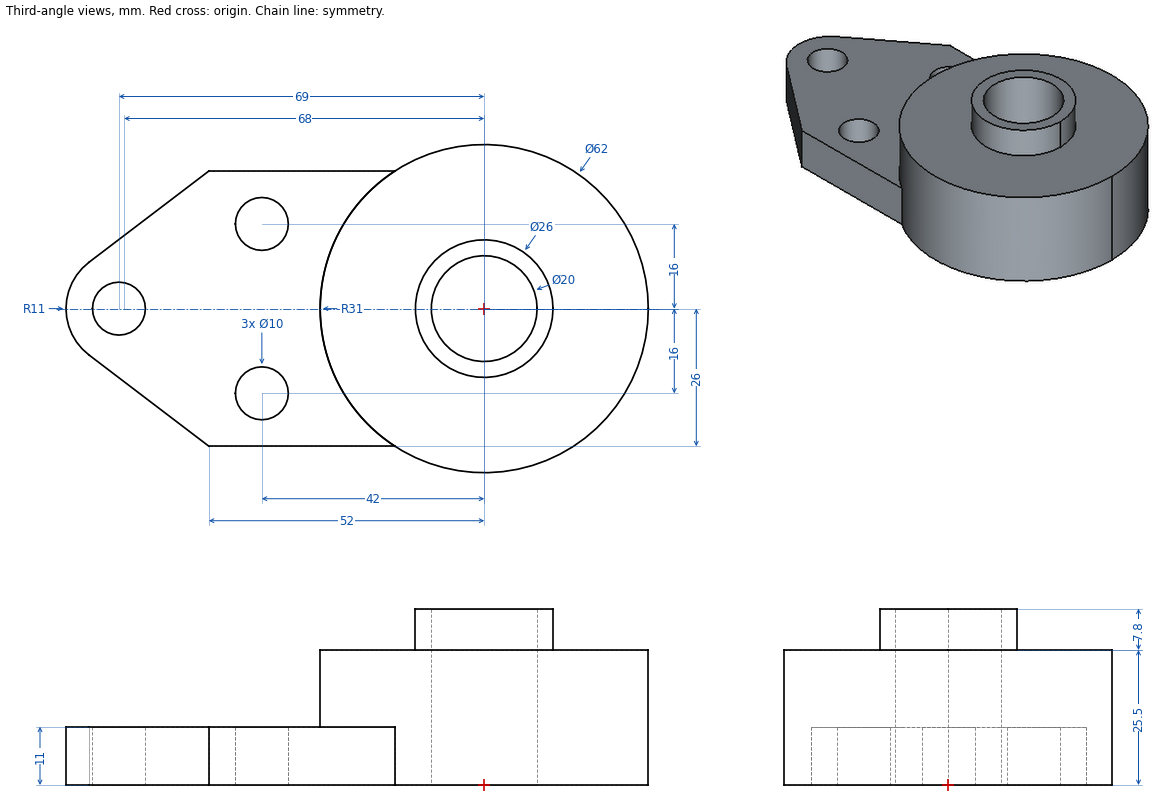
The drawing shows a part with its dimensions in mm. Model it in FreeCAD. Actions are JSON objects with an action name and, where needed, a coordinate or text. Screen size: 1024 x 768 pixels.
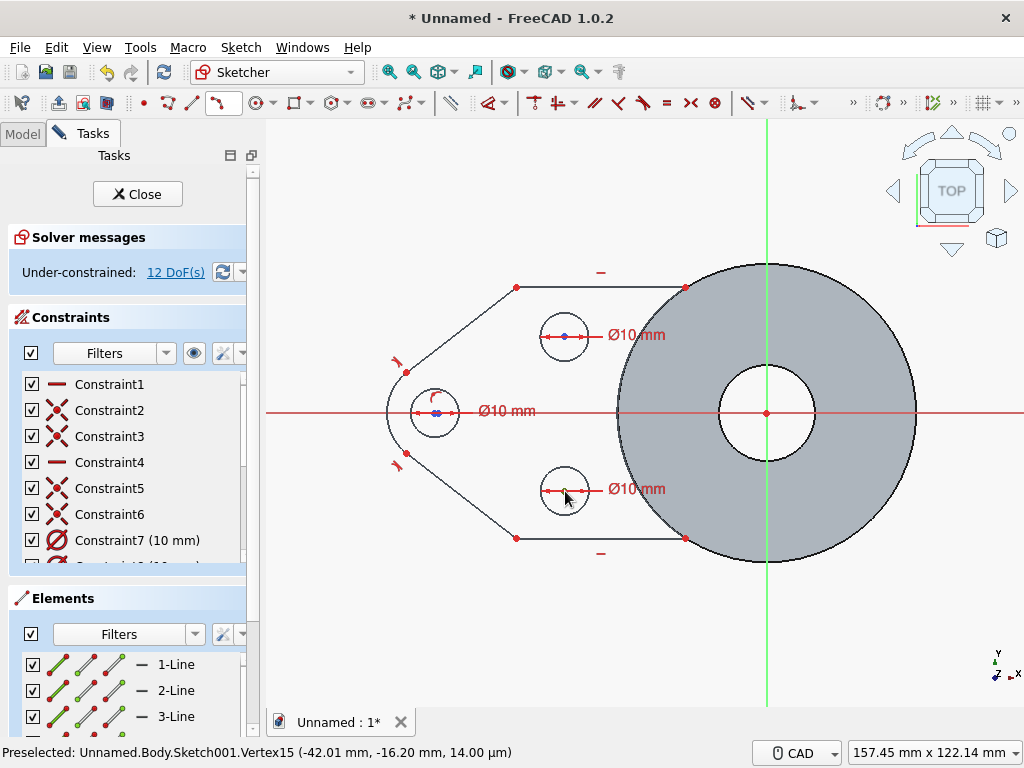
{"action": "left_click", "coordinate": [564, 337]}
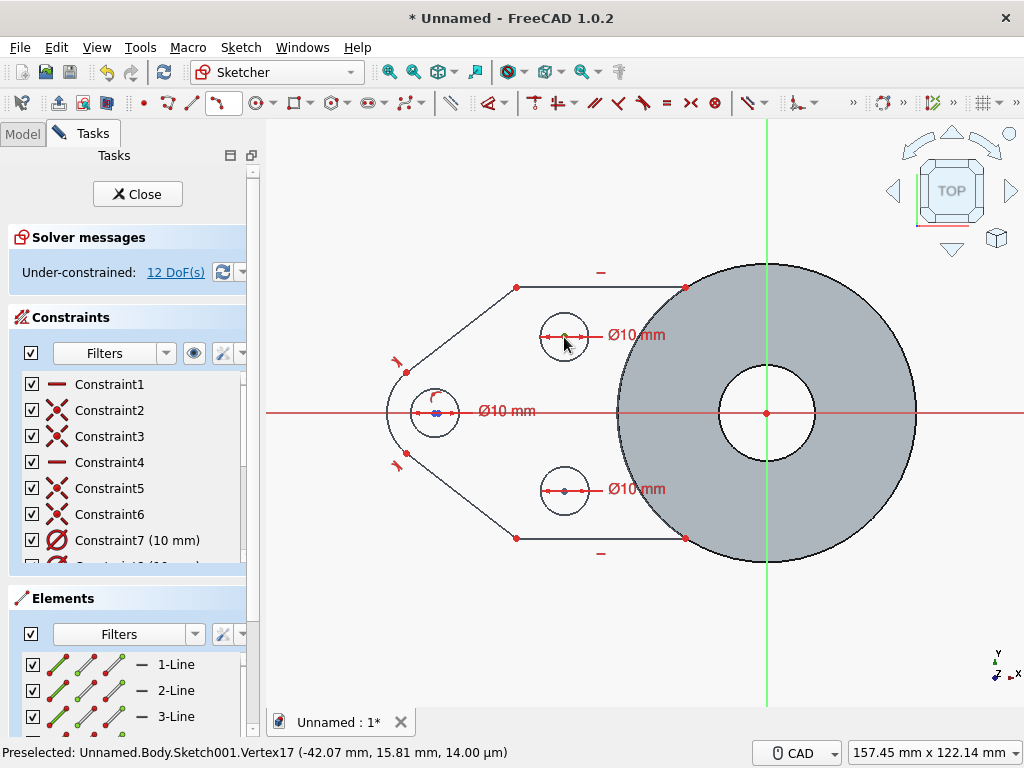
{"action": "key", "text": "v"}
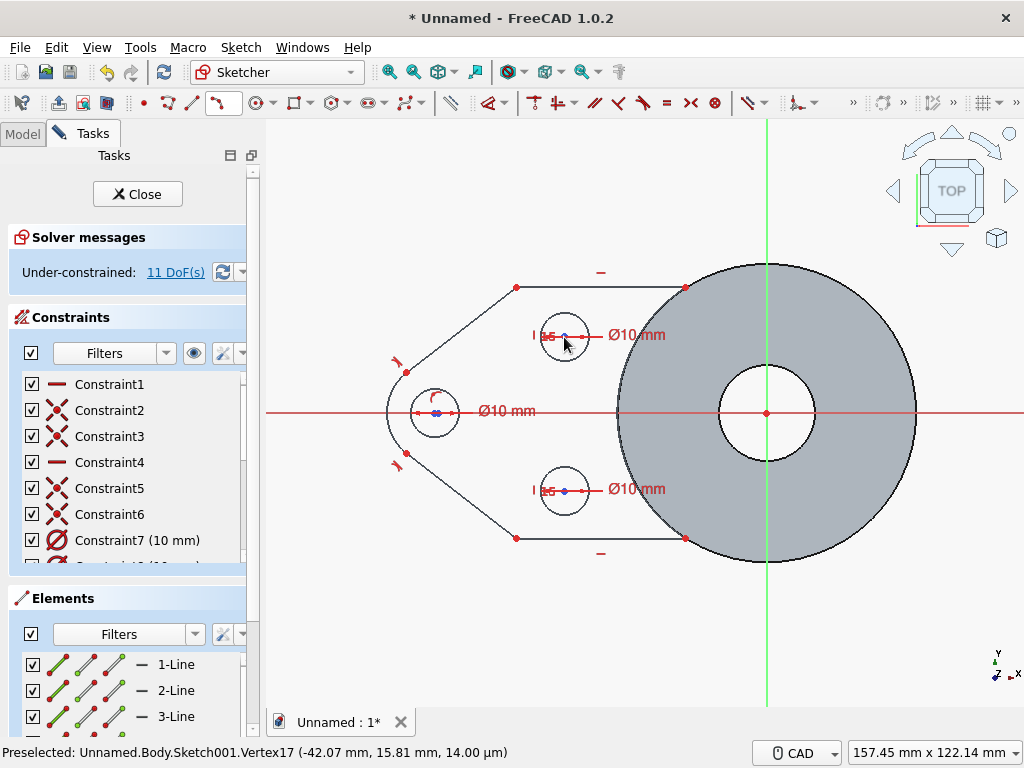
{"action": "left_click", "coordinate": [516, 539]}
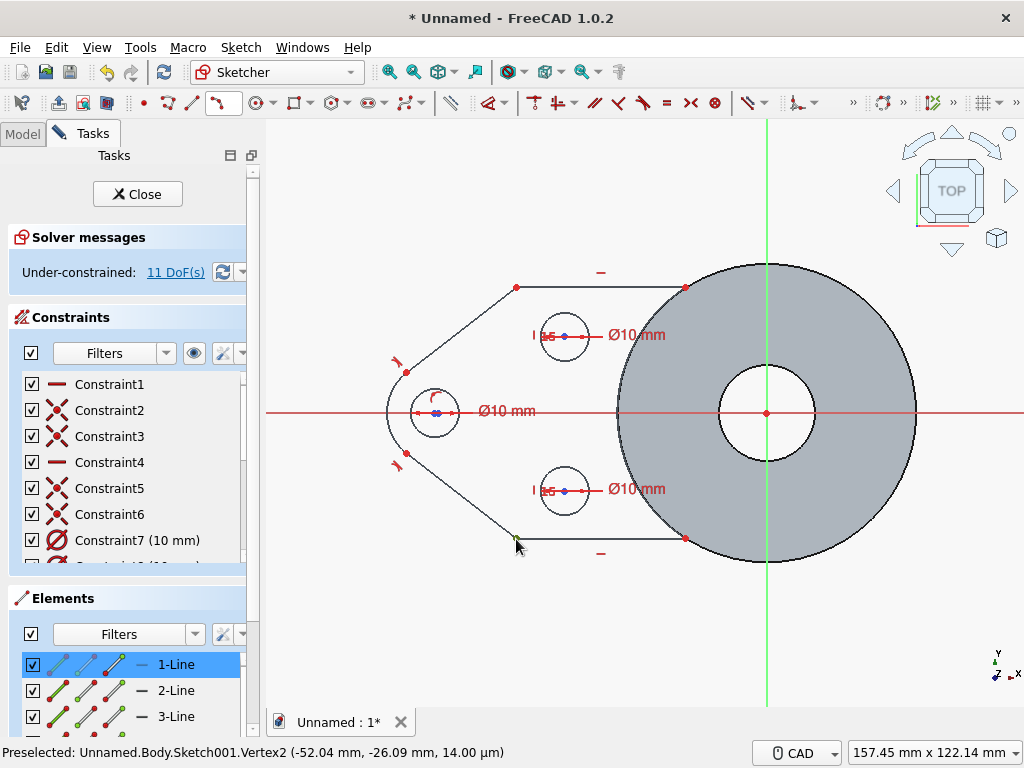
{"action": "left_click", "coordinate": [516, 287]}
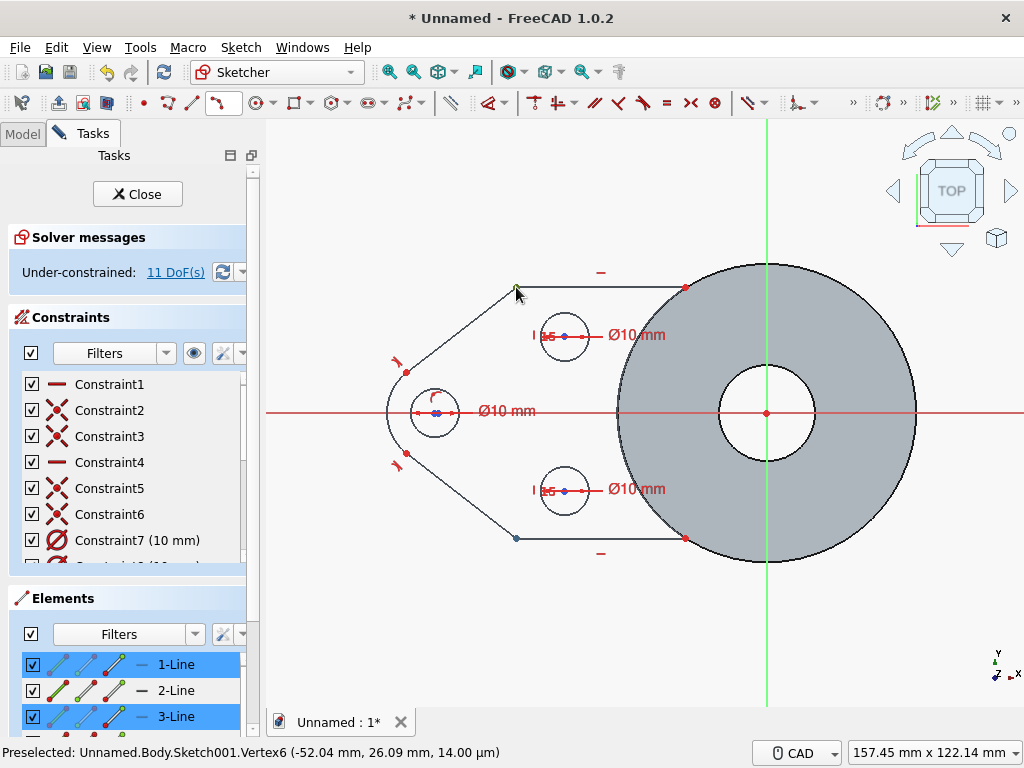
{"action": "left_click", "coordinate": [334, 413]}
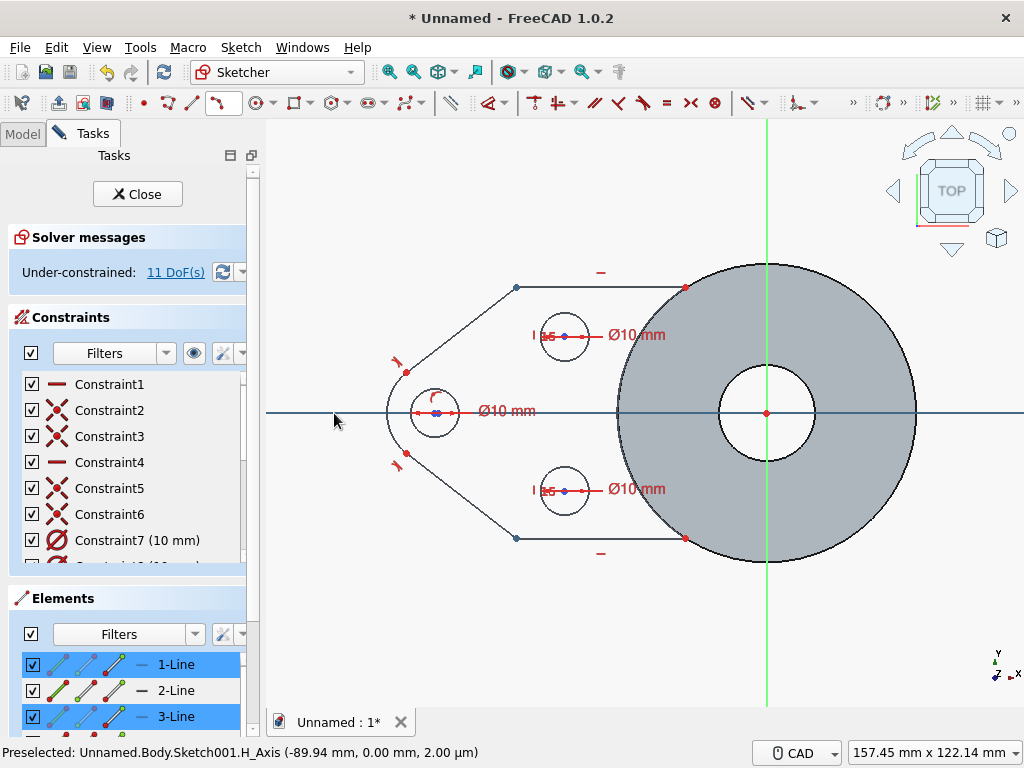
{"action": "key", "text": "s"}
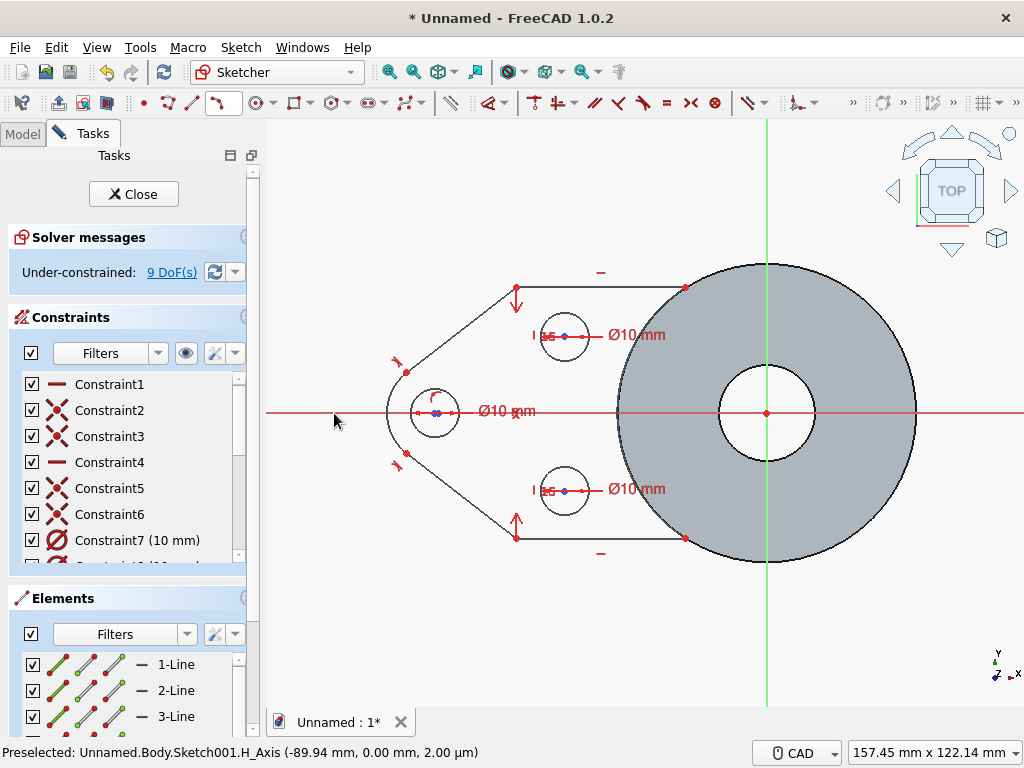
{"action": "key", "text": "d"}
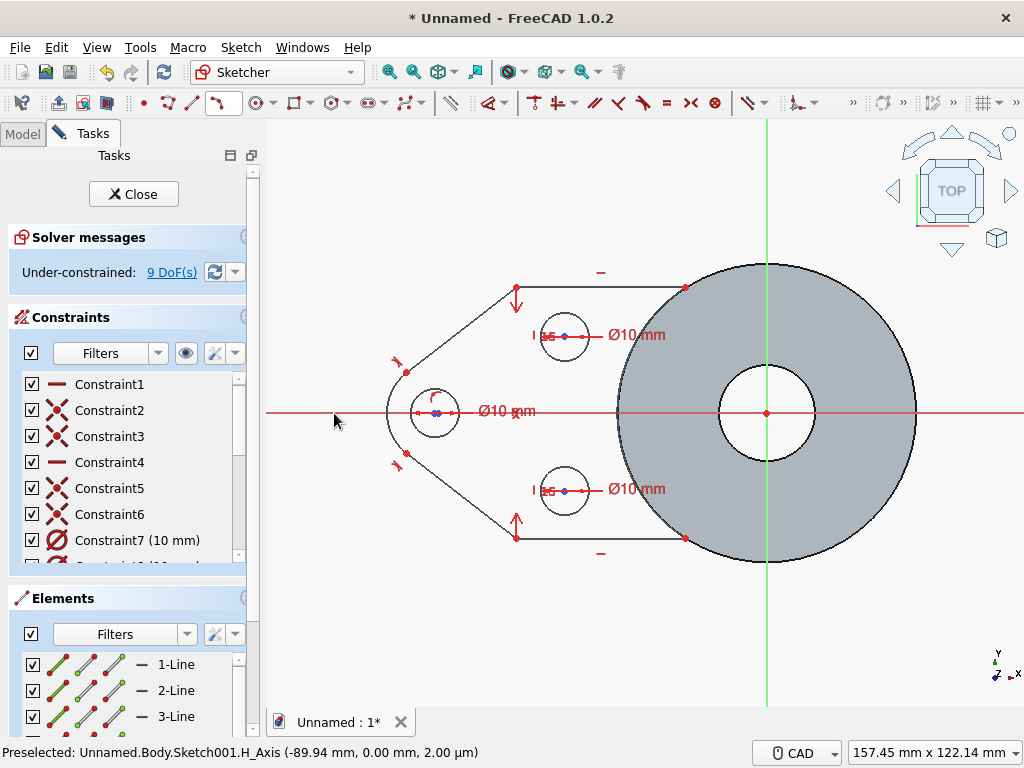
{"action": "left_click", "coordinate": [390, 395]}
{"action": "left_click", "coordinate": [360, 384]}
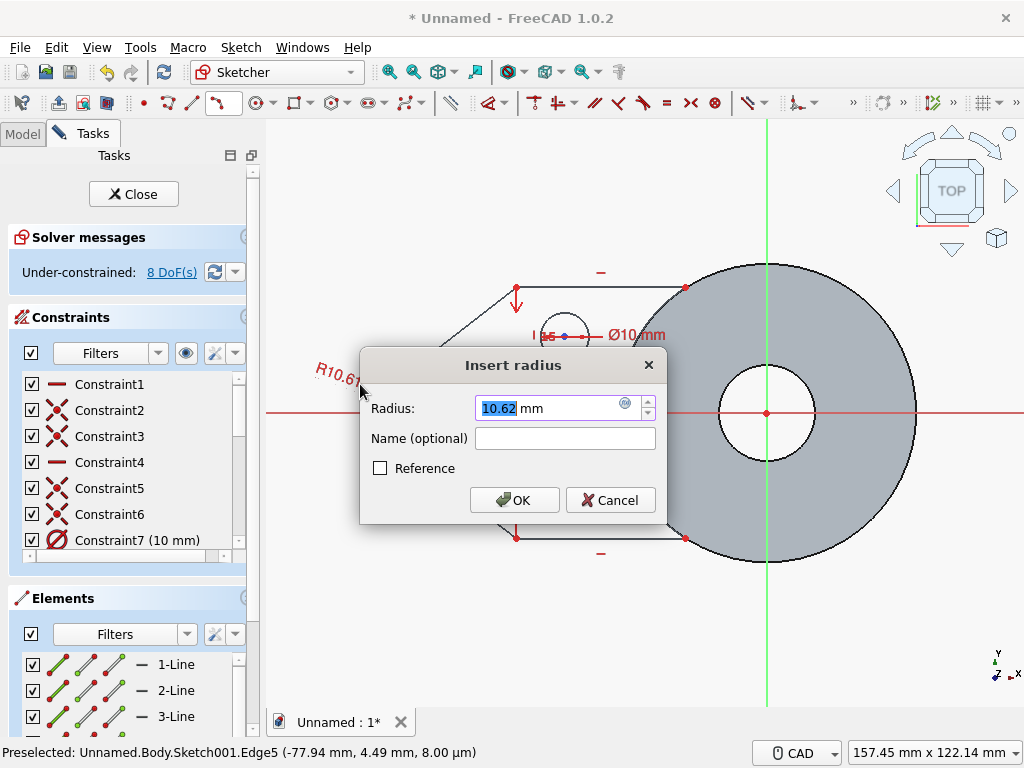
{"action": "type", "text": "11"}
{"action": "key", "text": "Return"}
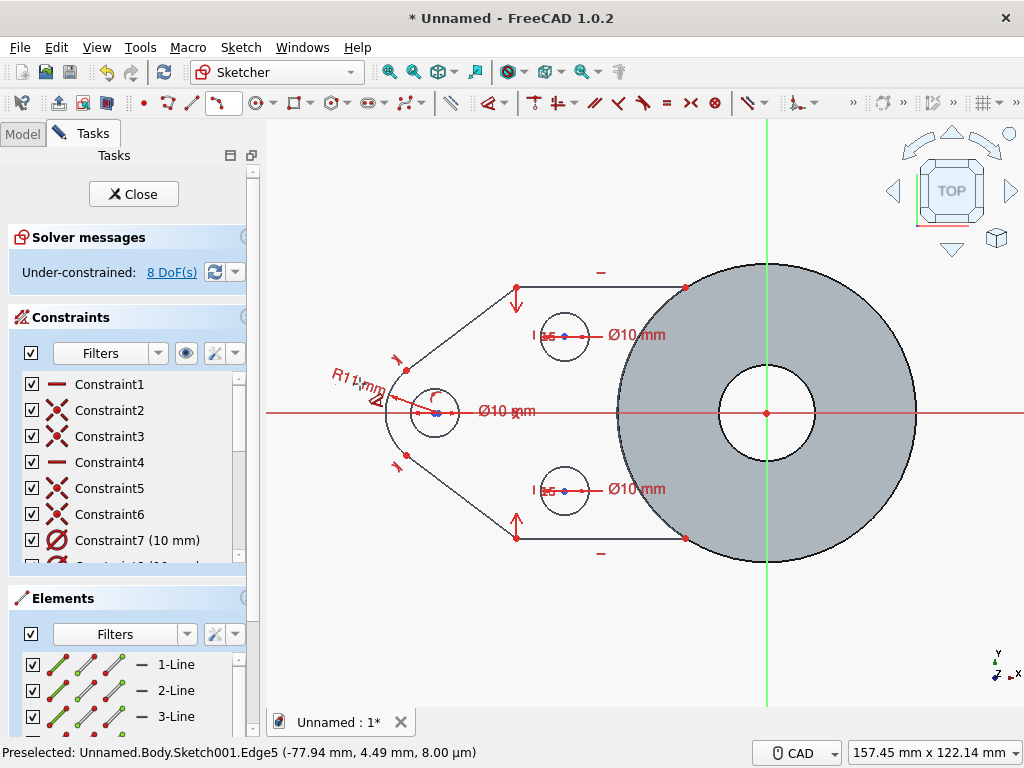
{"action": "left_click", "coordinate": [629, 355]}
{"action": "left_click", "coordinate": [654, 271]}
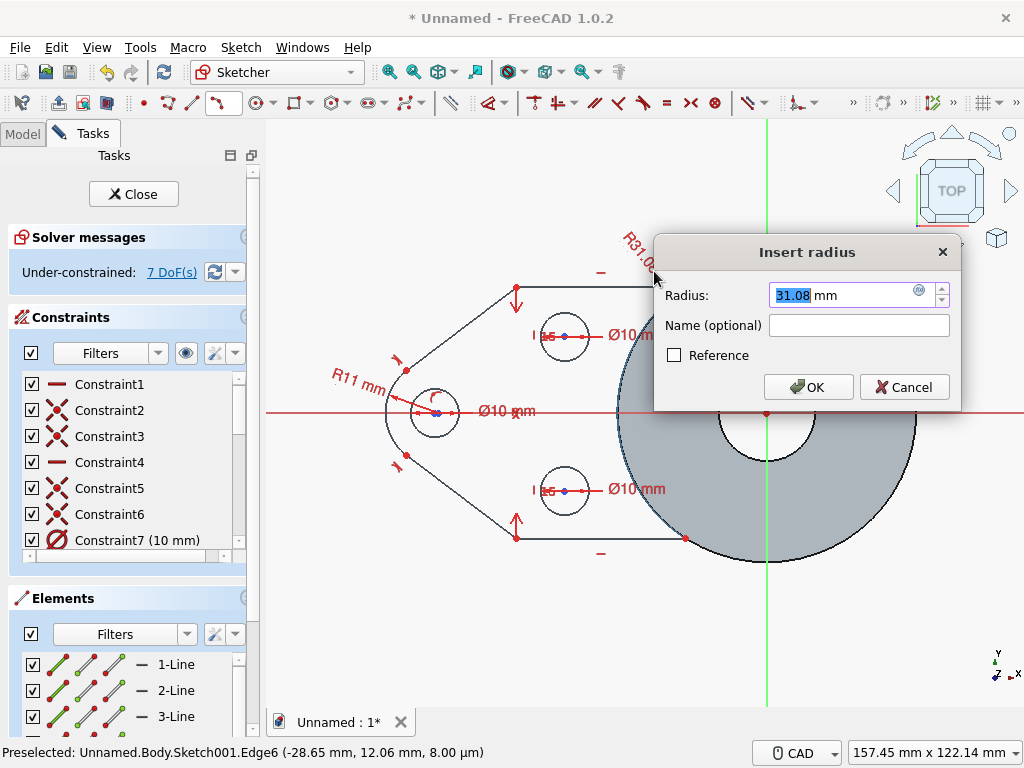
{"action": "type", "text": "31"}
{"action": "key", "text": "Return"}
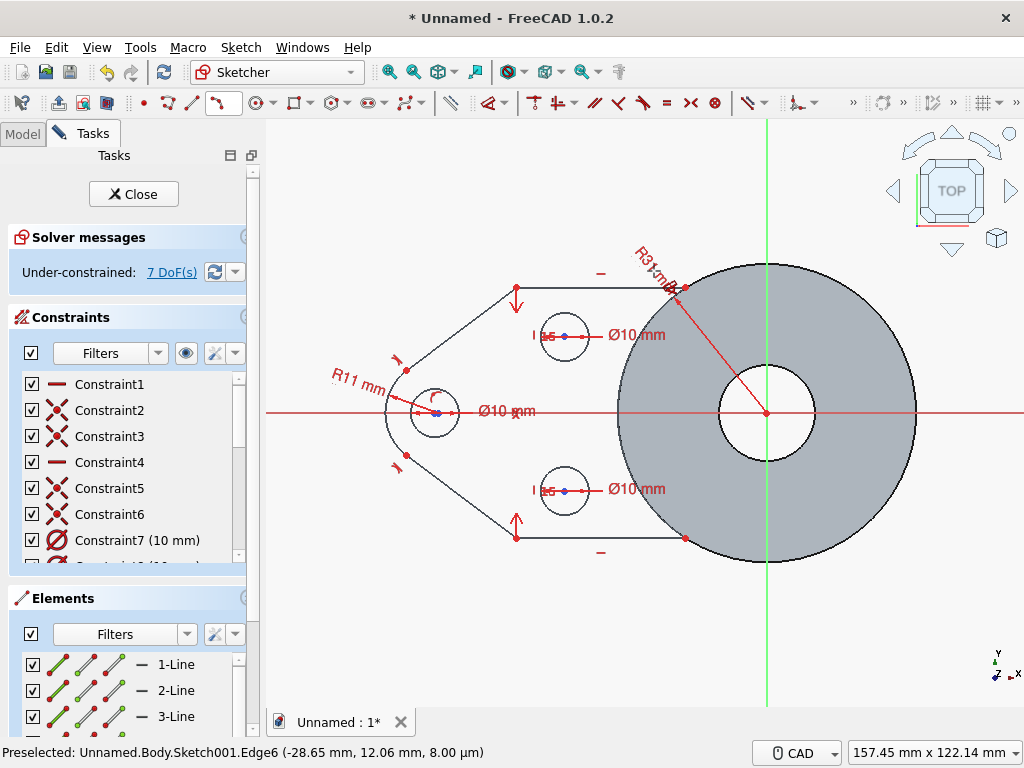
{"action": "left_click", "coordinate": [565, 491]}
{"action": "left_click", "coordinate": [619, 525]}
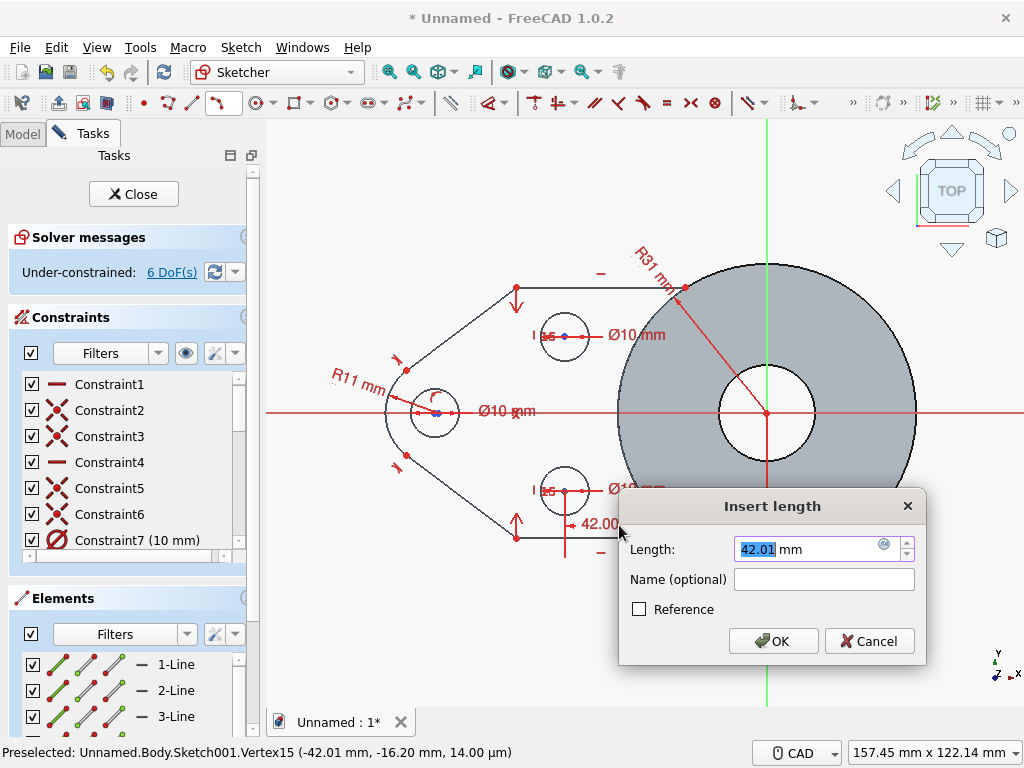
{"action": "type", "text": "42"}
{"action": "key", "text": "Return"}